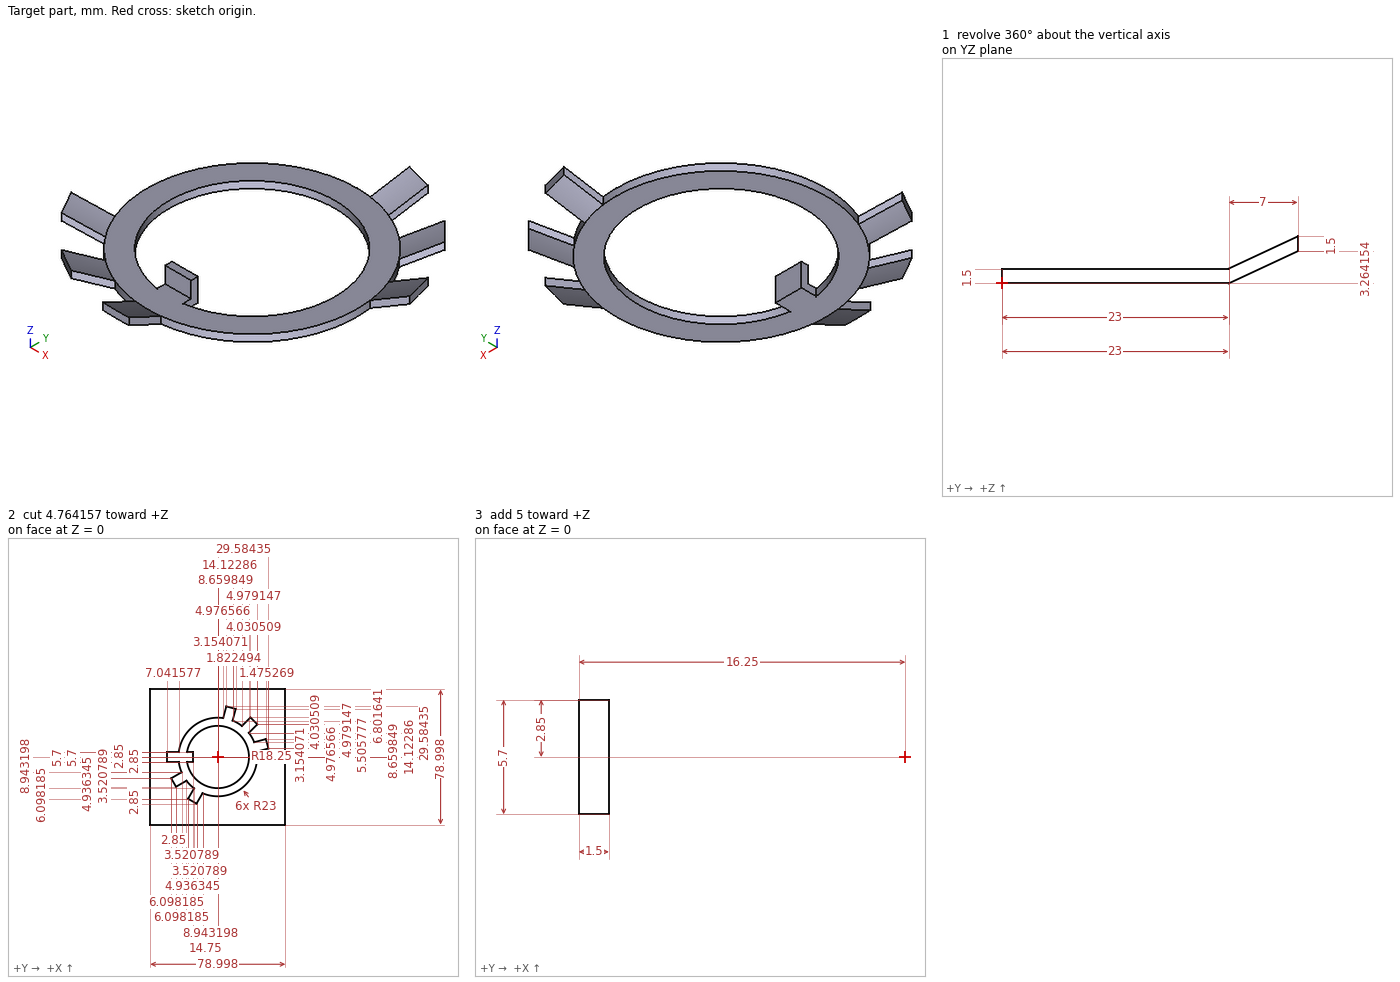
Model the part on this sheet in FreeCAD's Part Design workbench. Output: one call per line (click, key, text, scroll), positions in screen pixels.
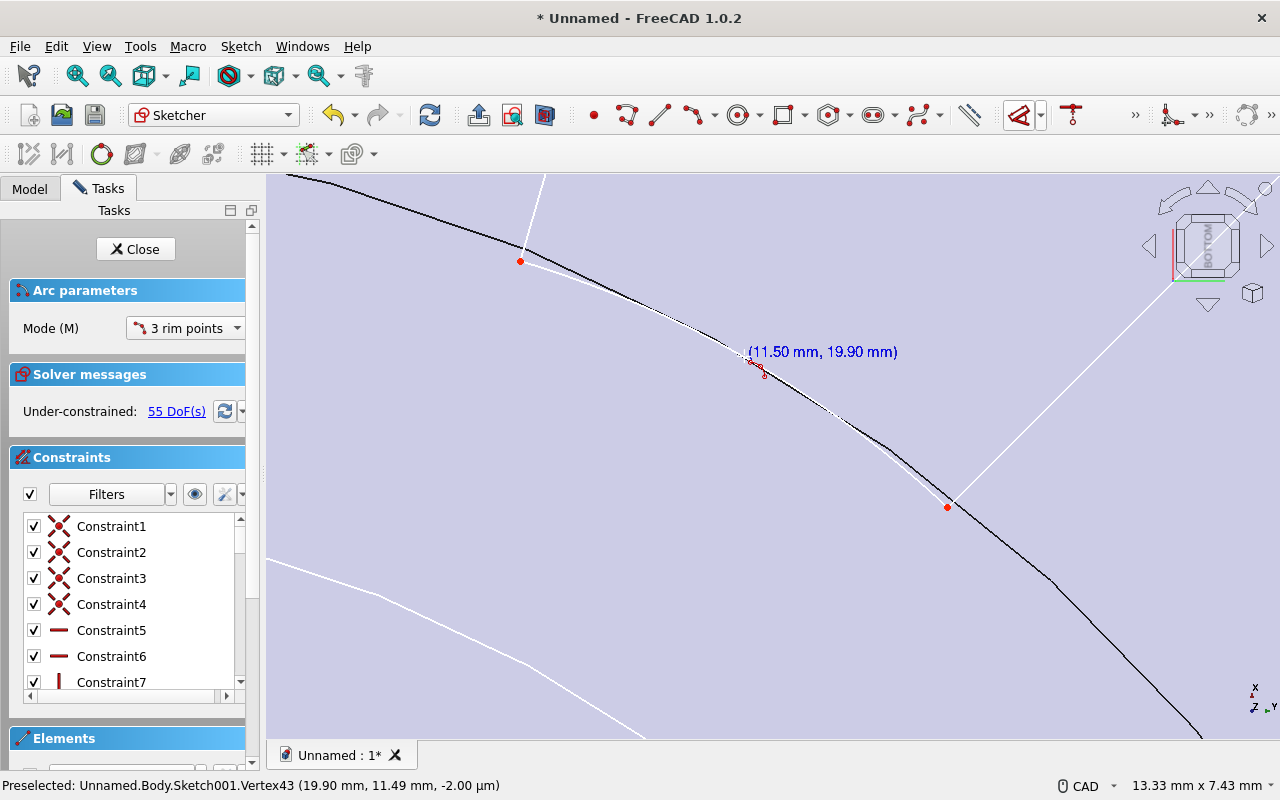
scroll(759, 365, down, 14)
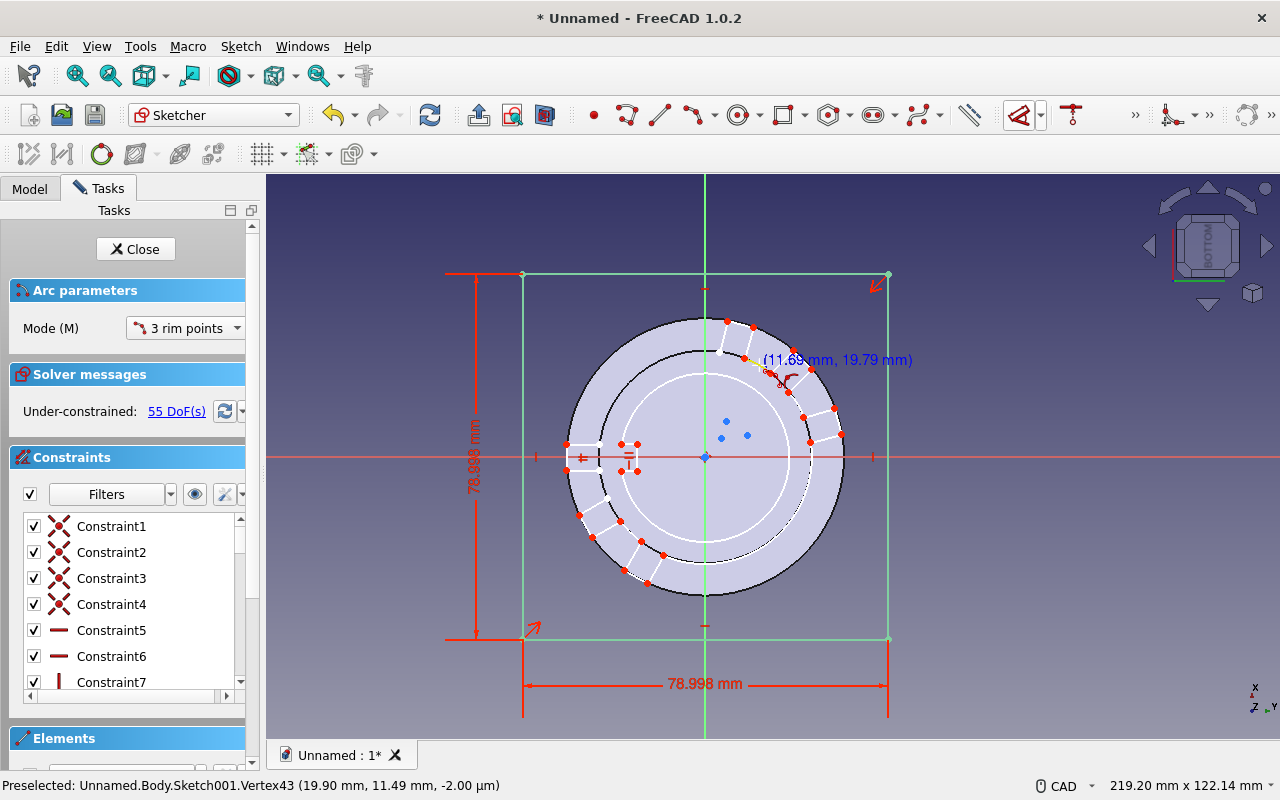
click(720, 353)
click(600, 445)
click(641, 372)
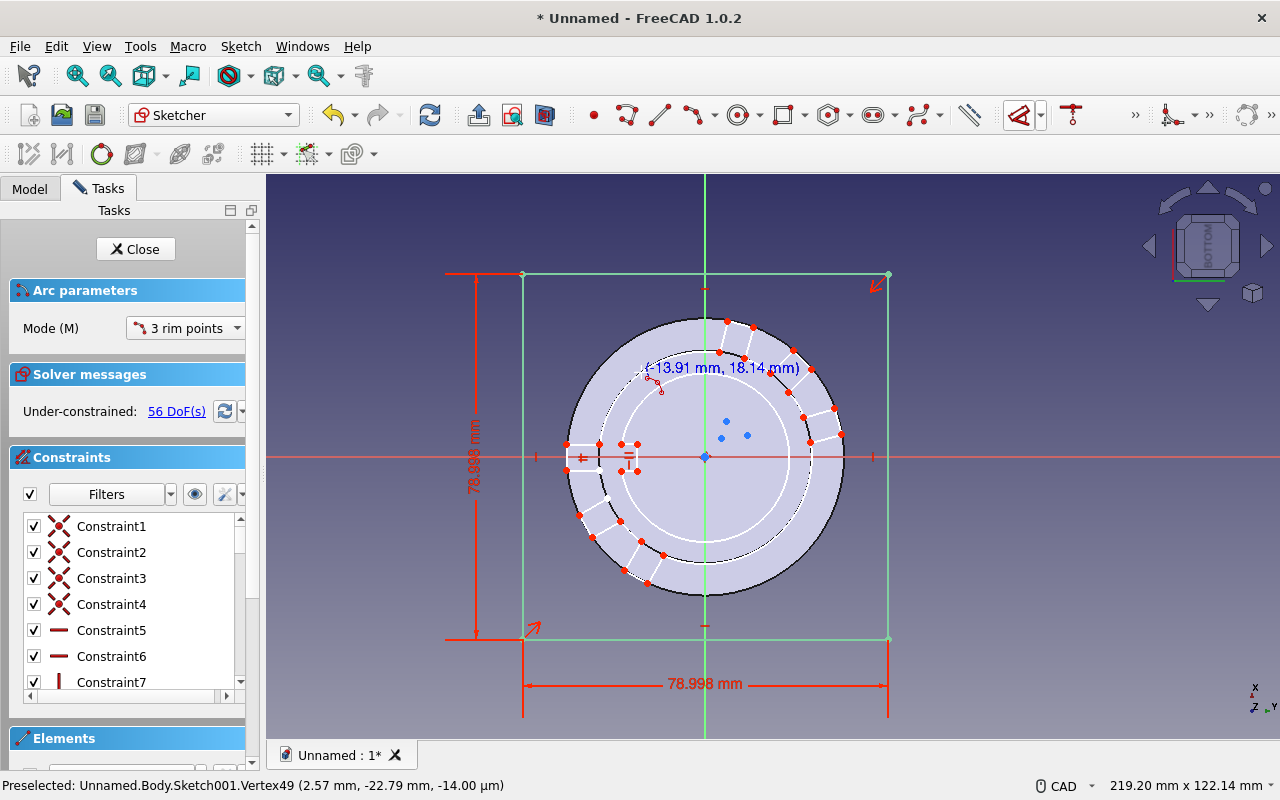
click(600, 471)
click(607, 499)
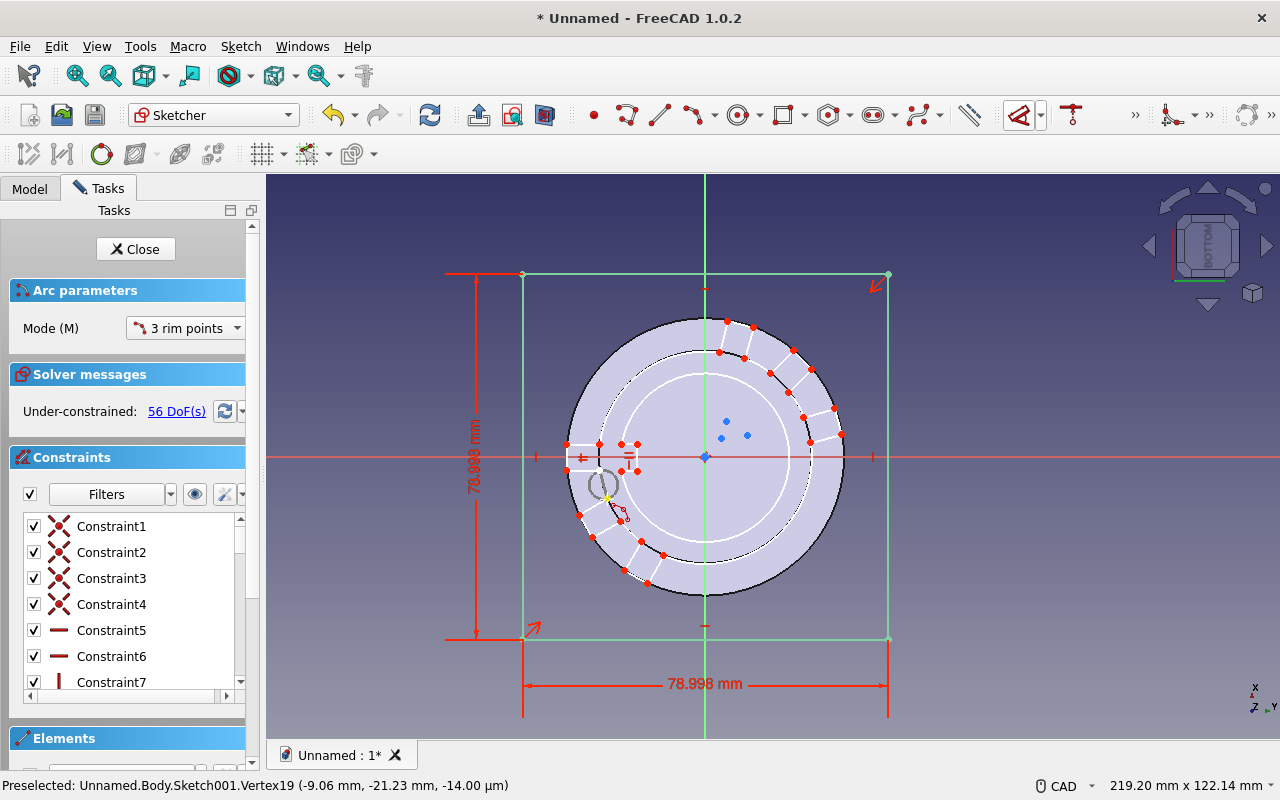
scroll(603, 484, up, 14)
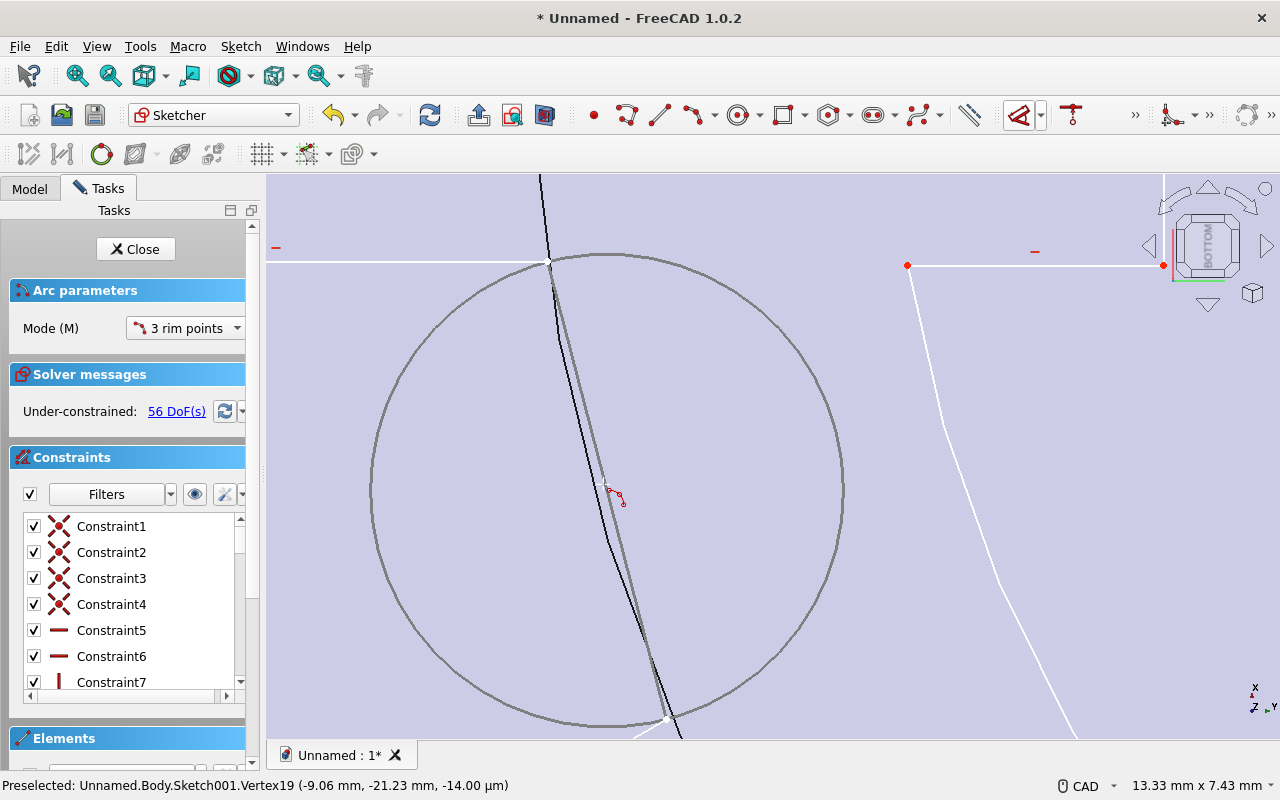
click(591, 483)
key(Escape)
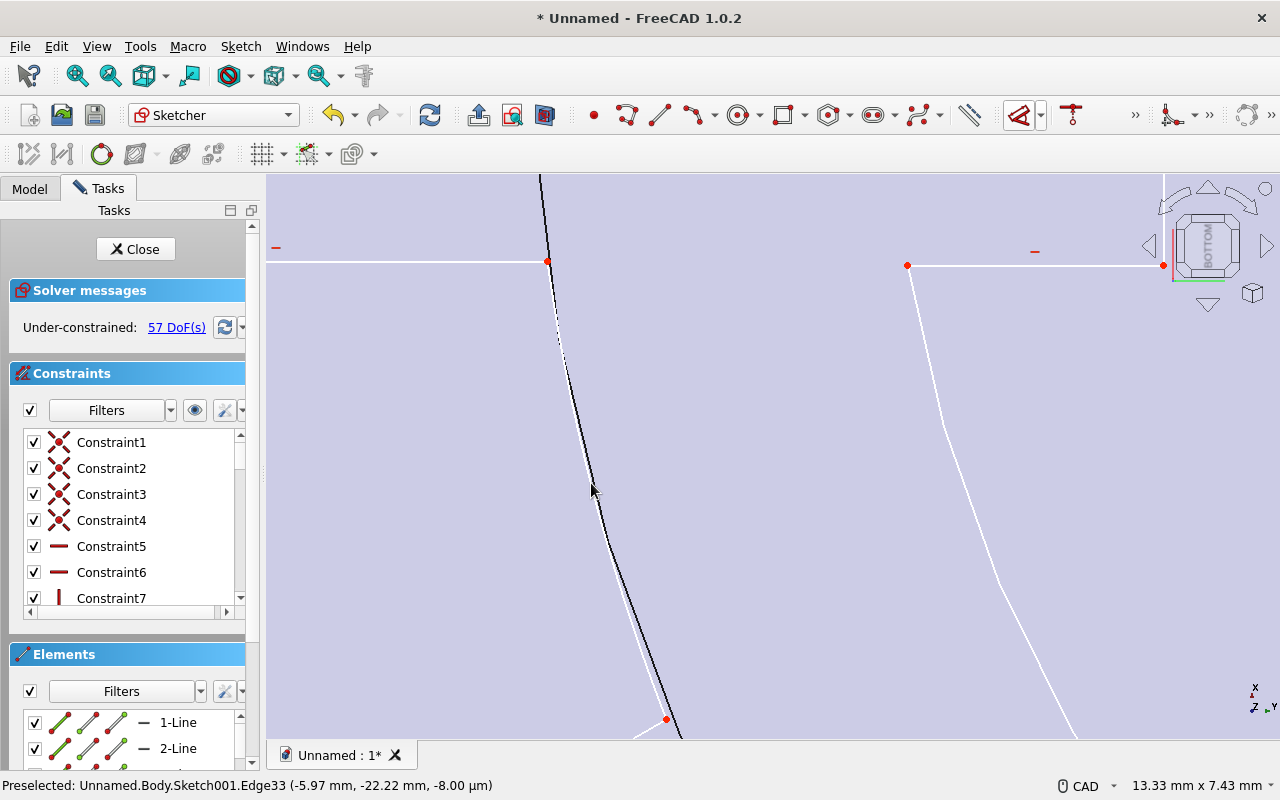
scroll(602, 484, down, 14)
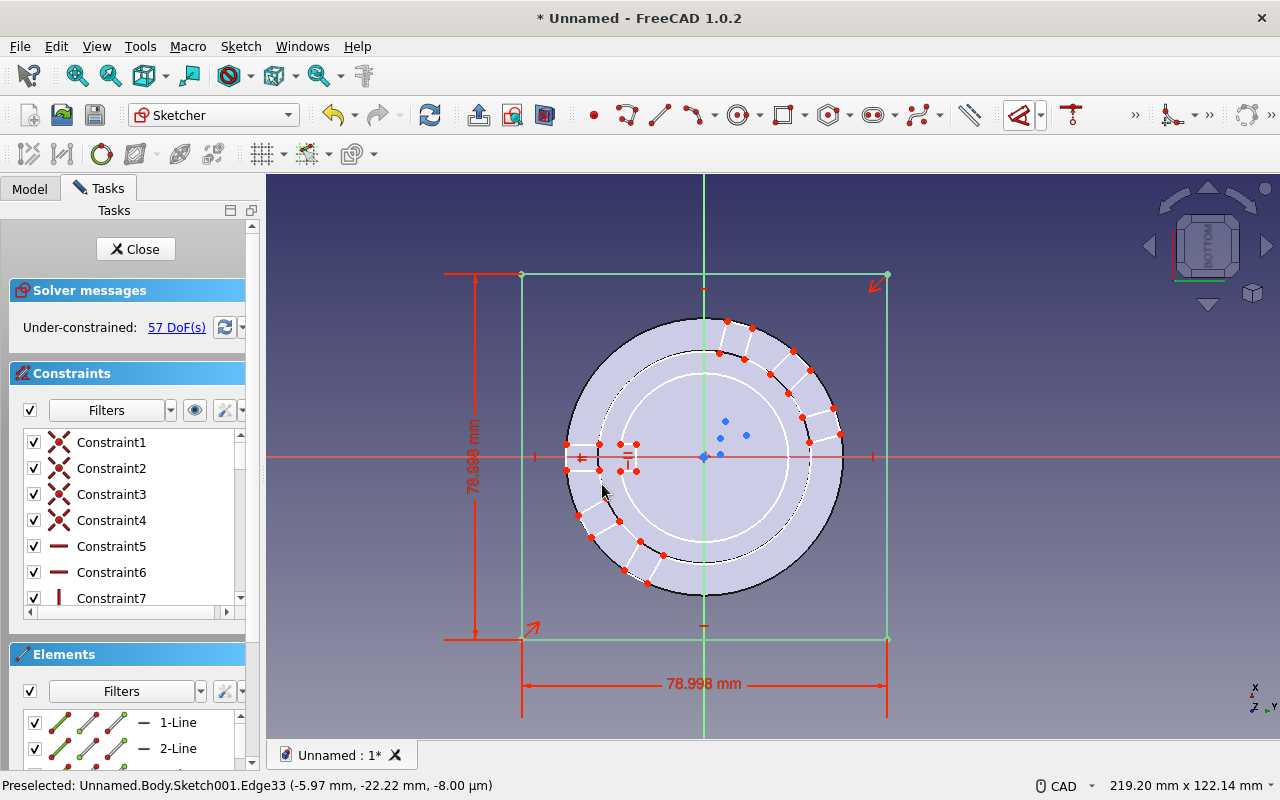
click(735, 536)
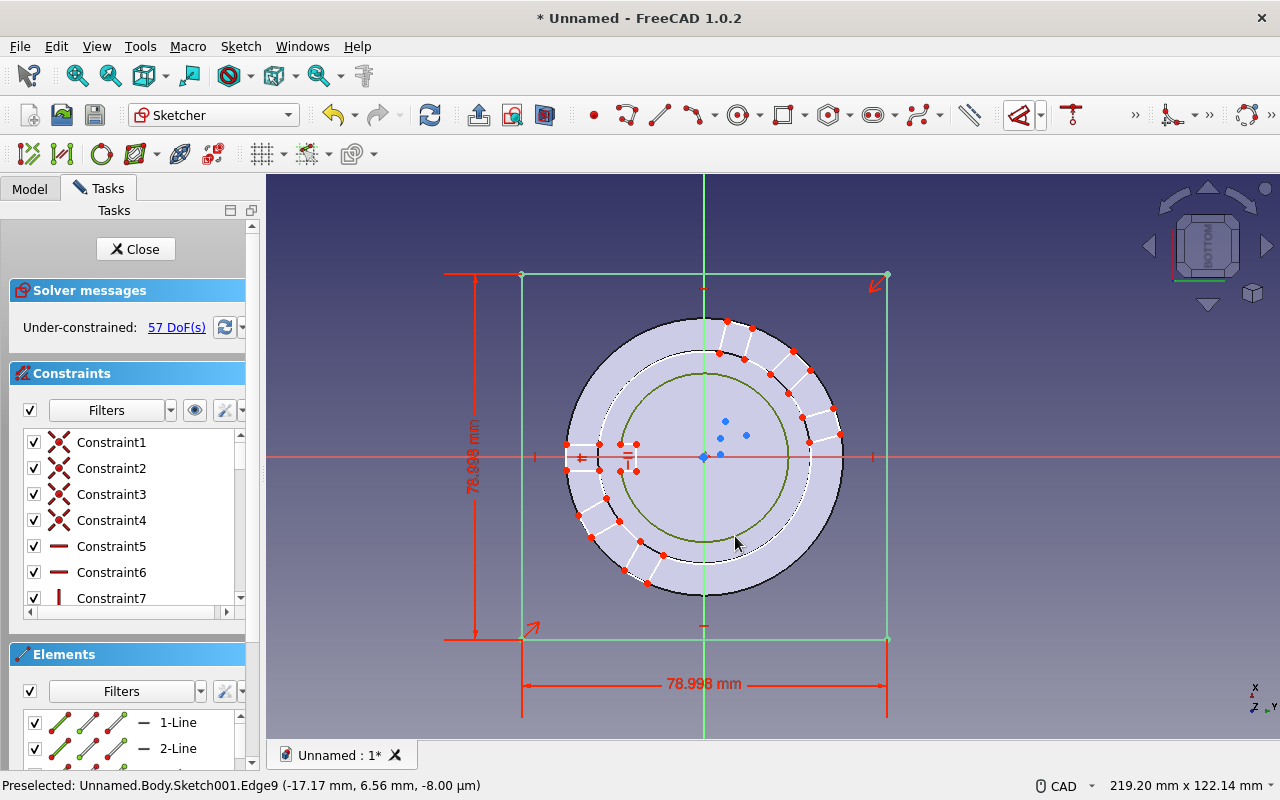
click(629, 532)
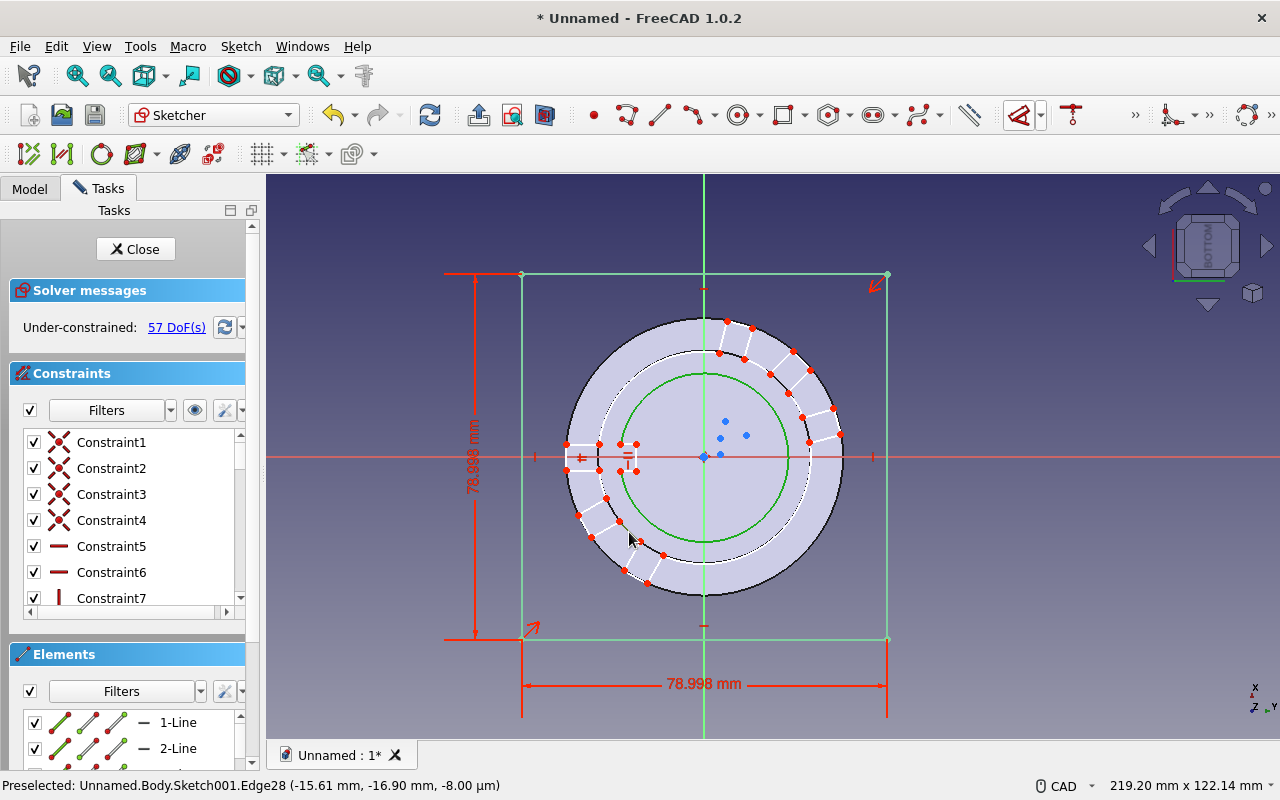
key(c)